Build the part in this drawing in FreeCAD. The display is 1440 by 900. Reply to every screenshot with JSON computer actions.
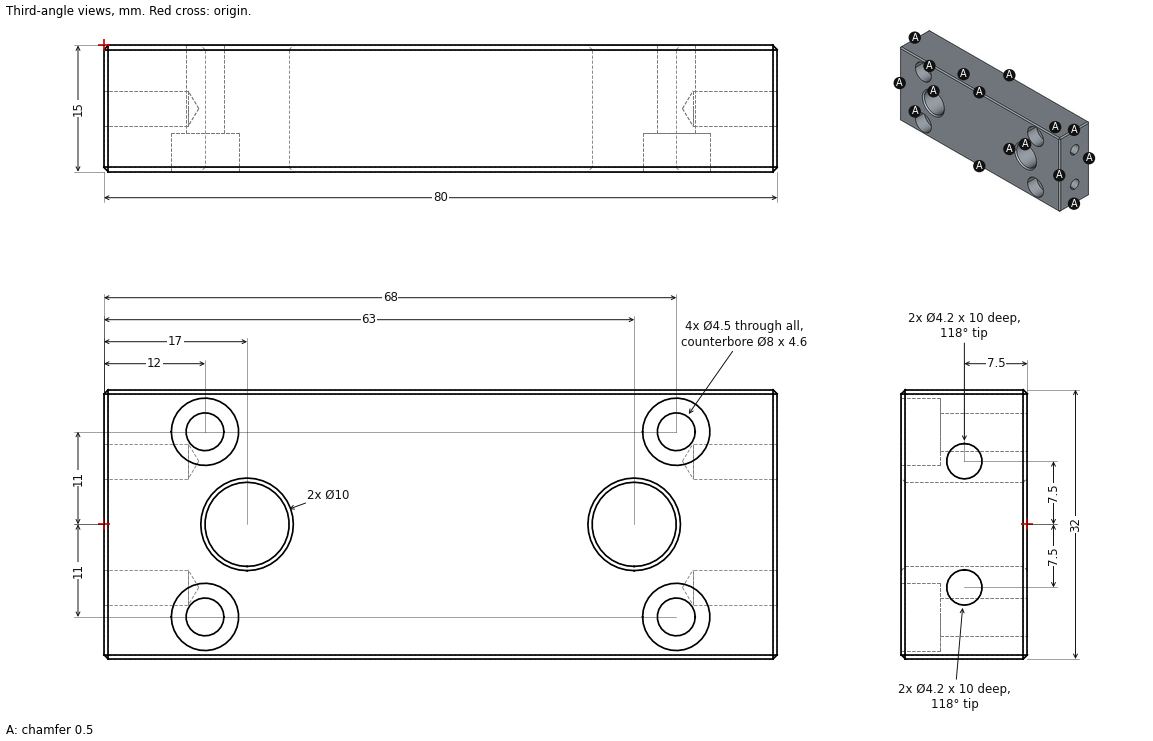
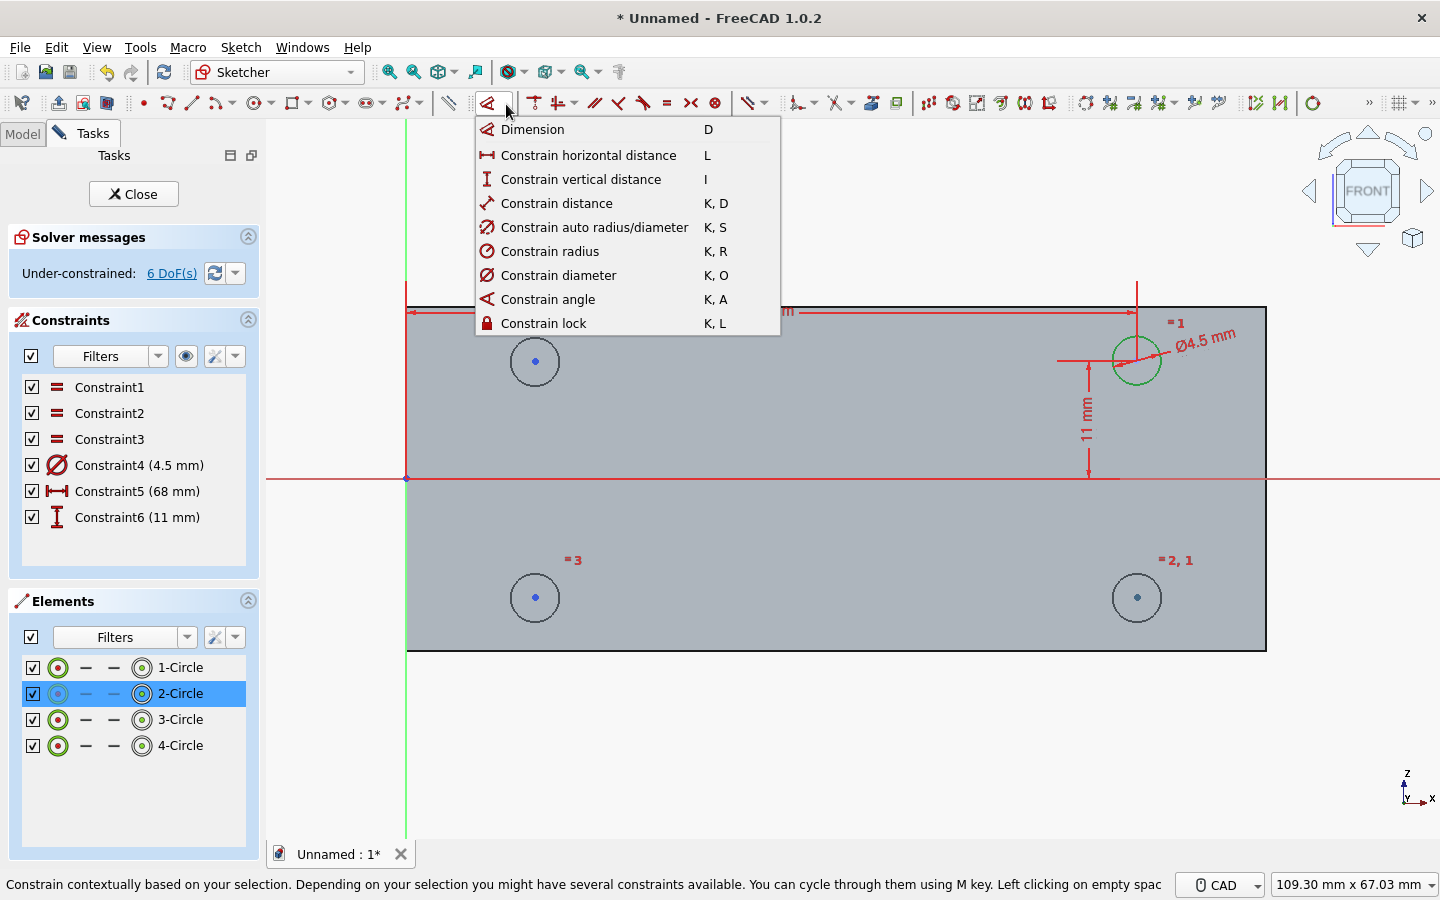
{"action": "left_click", "coordinate": [628, 155]}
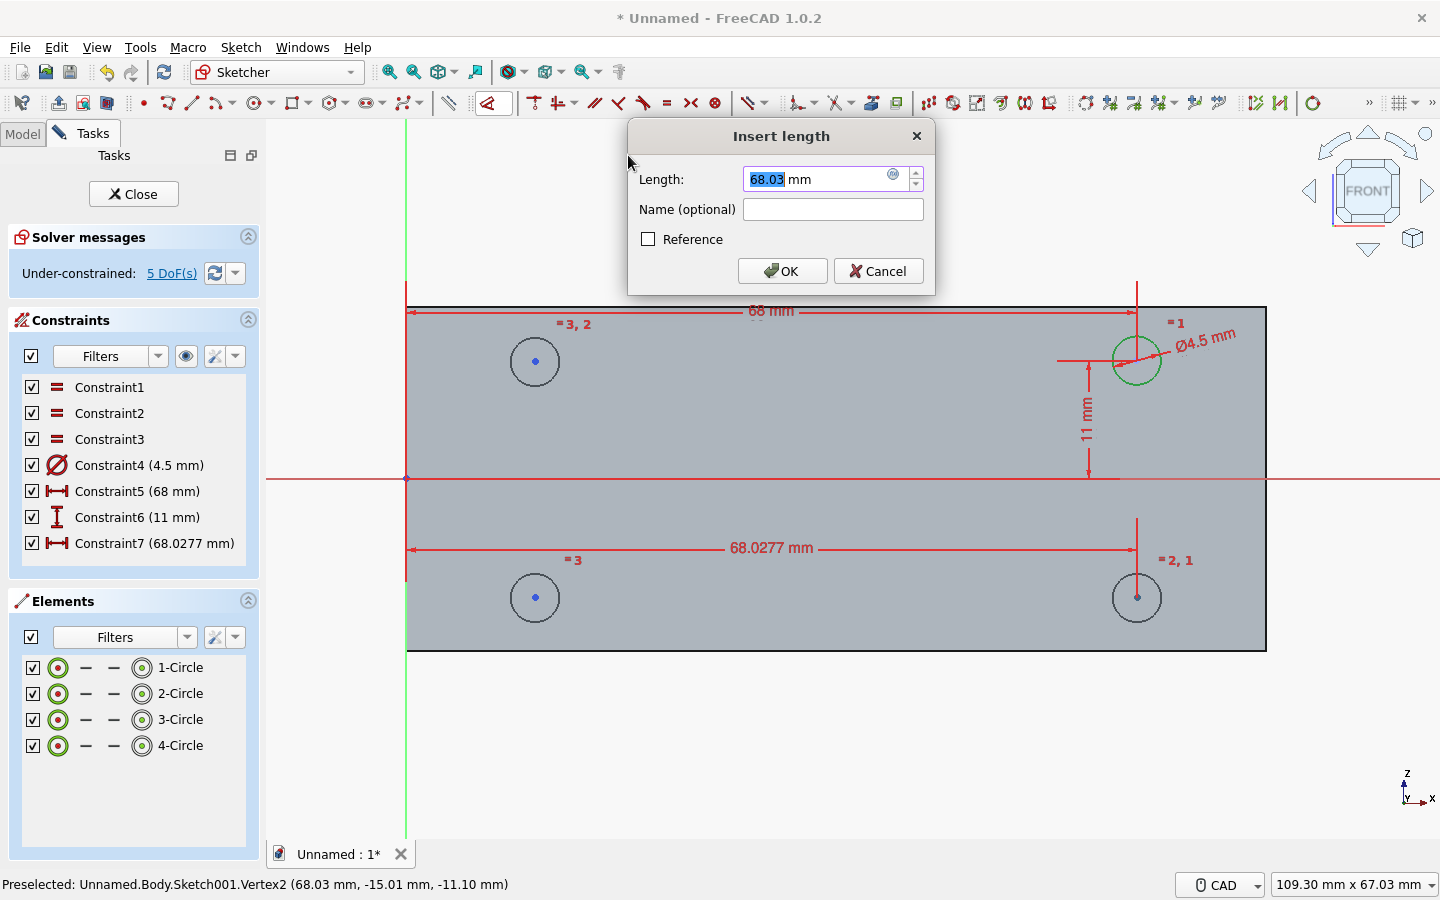
{"action": "type", "text": "68"}
{"action": "key", "text": "Return"}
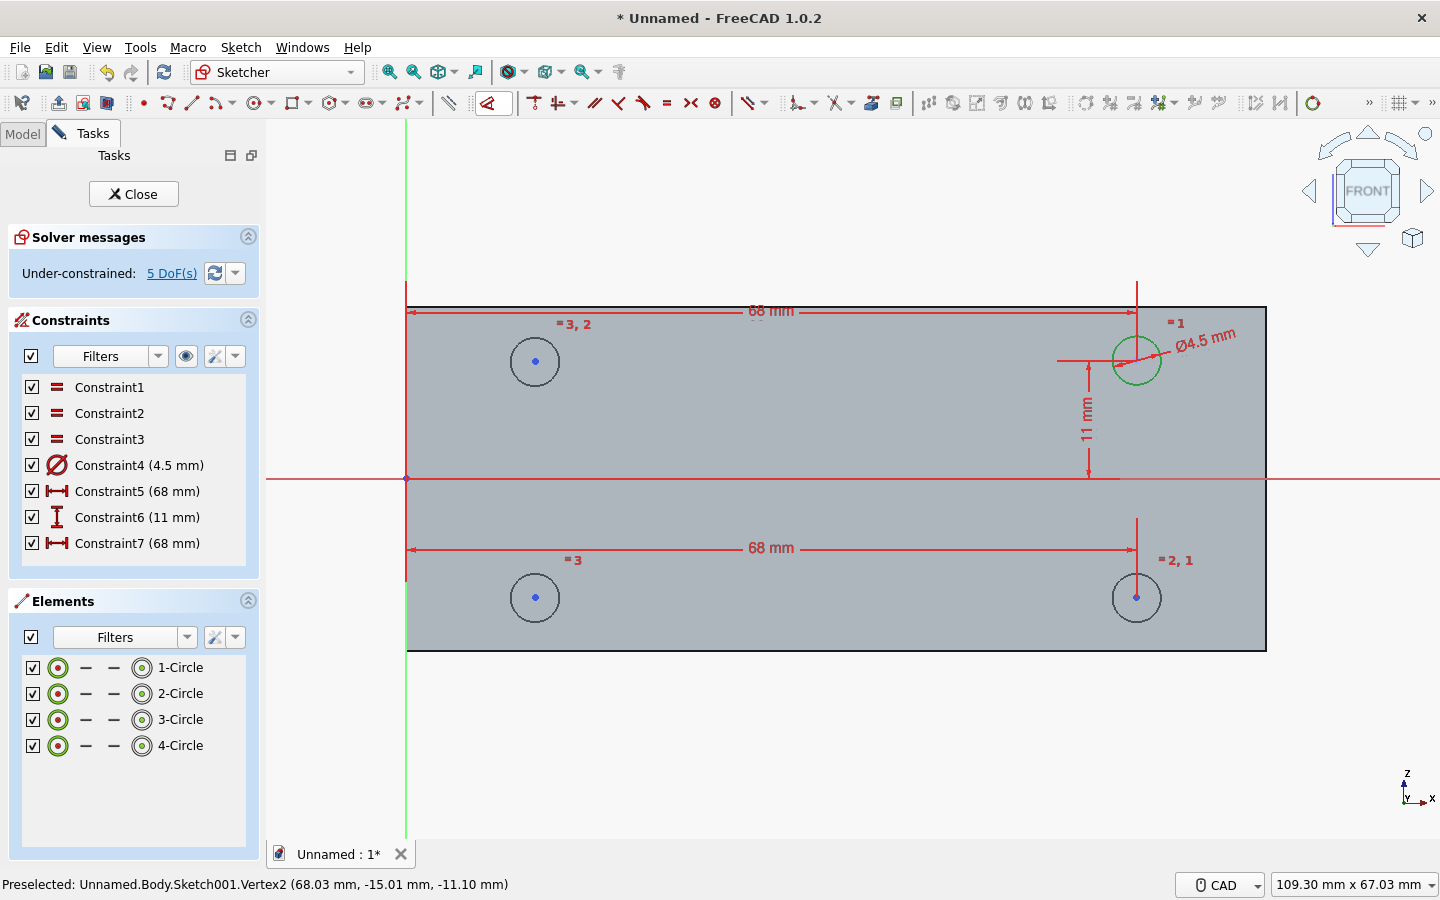
{"action": "left_click", "coordinate": [1137, 598]}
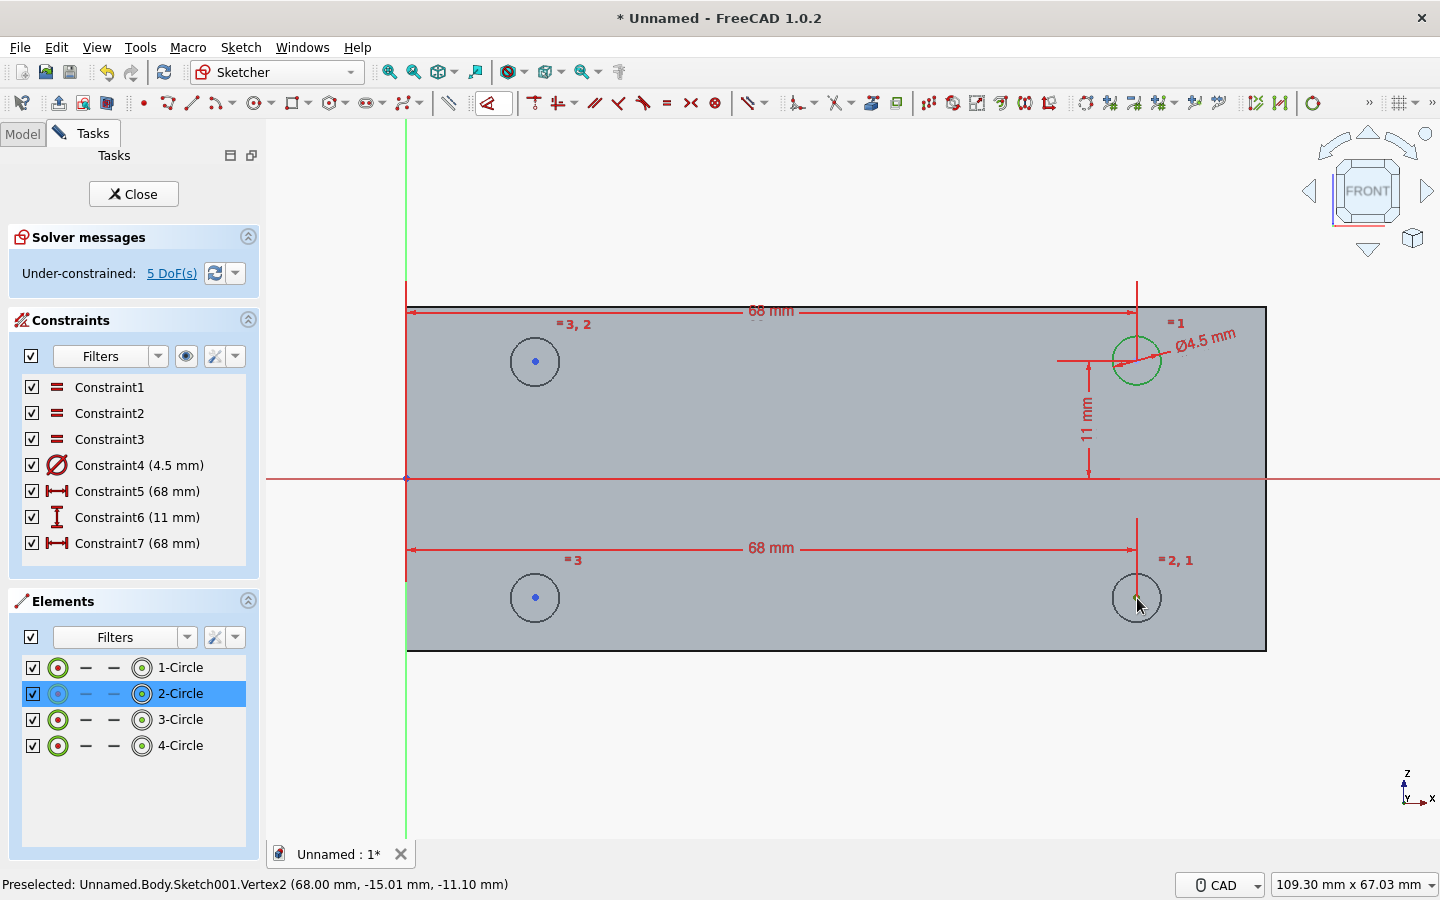
{"action": "left_click", "coordinate": [506, 104]}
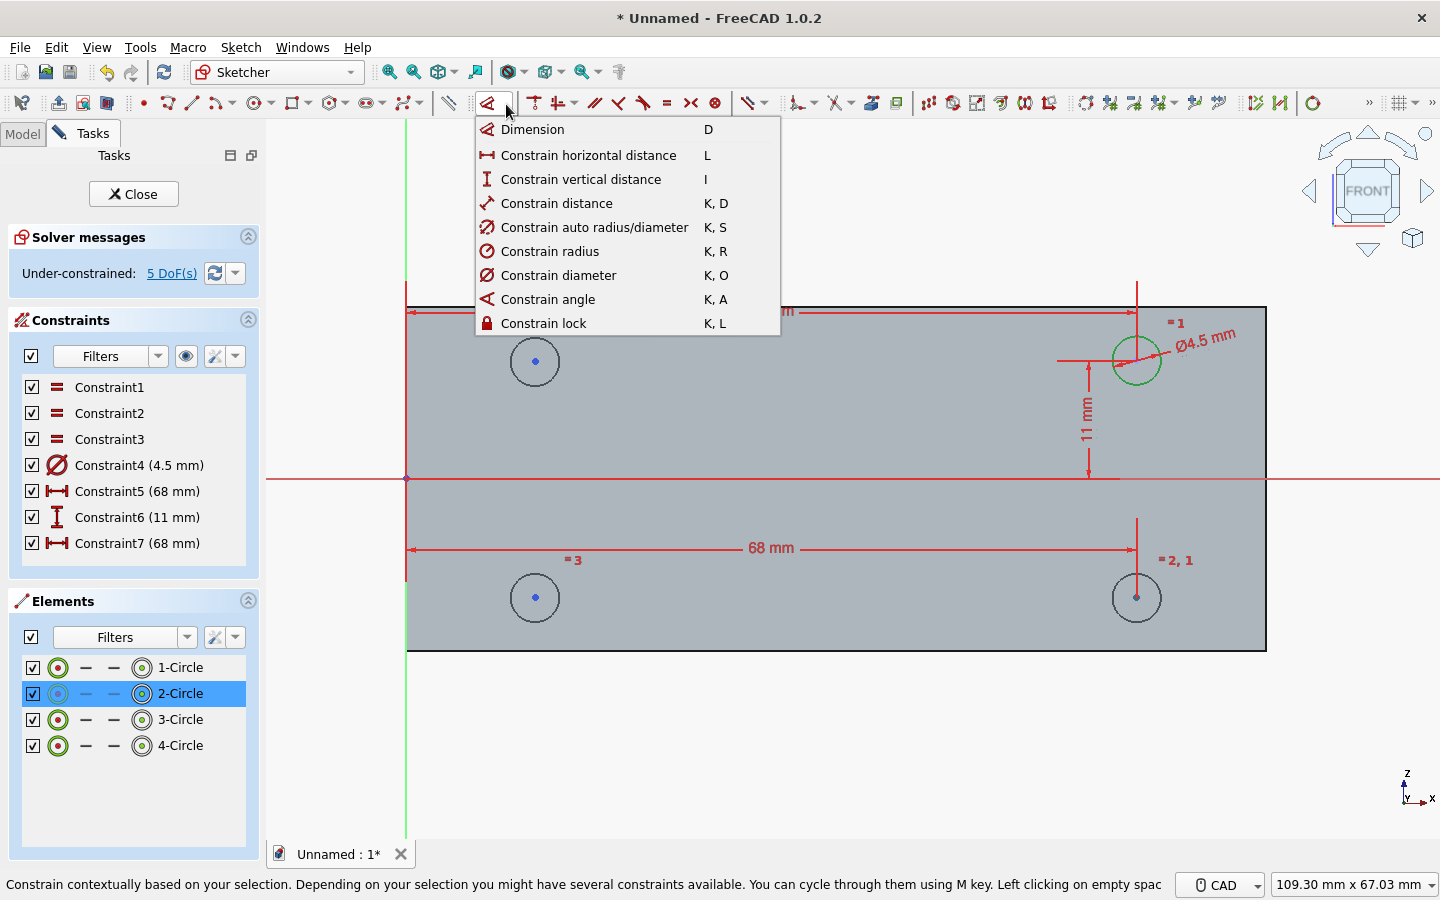
{"action": "left_click", "coordinate": [628, 179]}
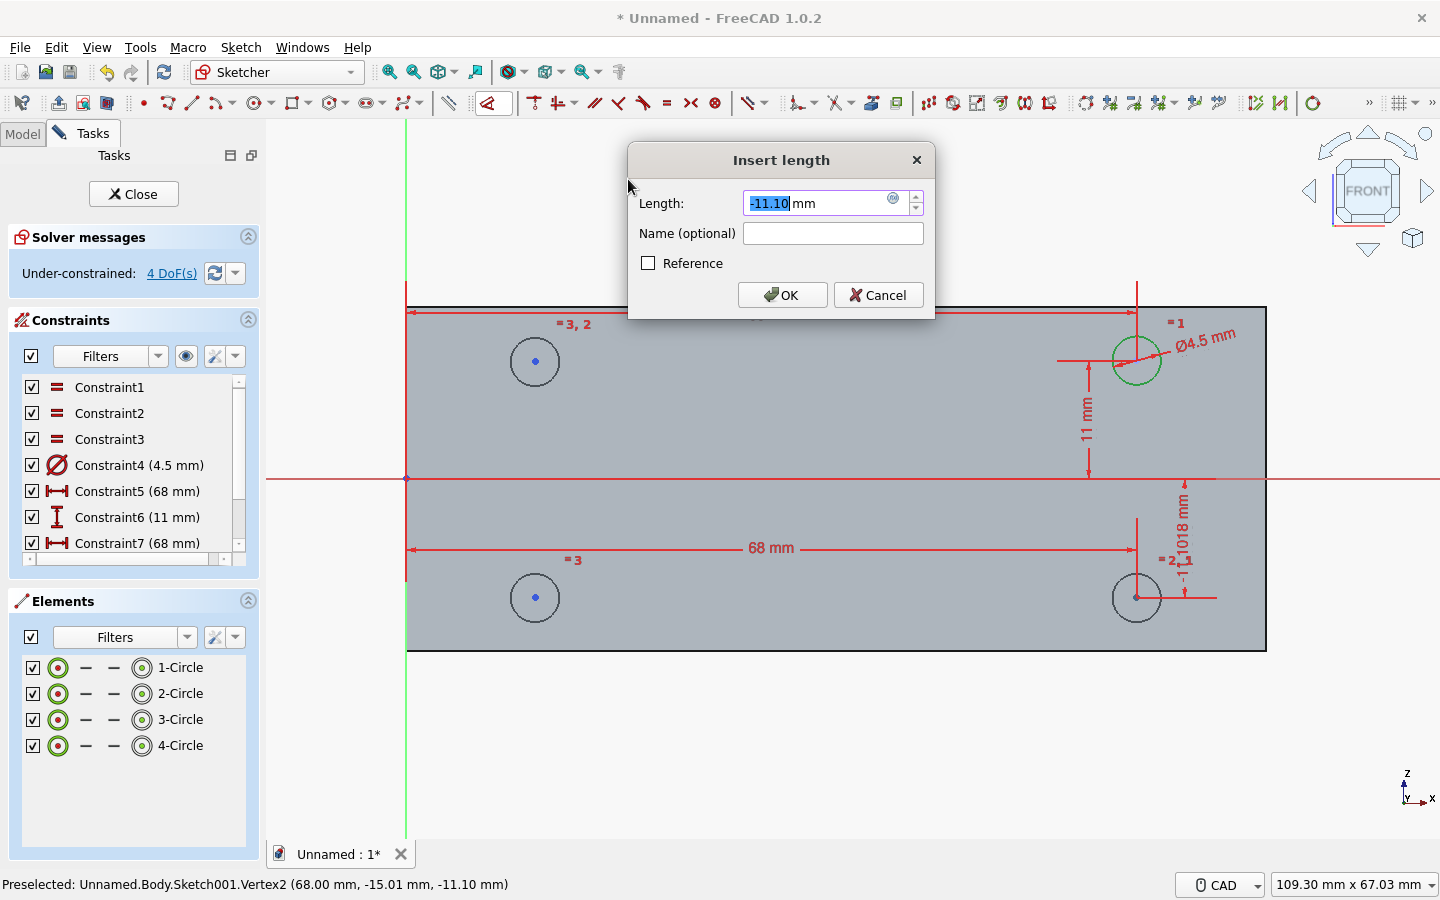
{"action": "type", "text": "-11"}
{"action": "key", "text": "Return"}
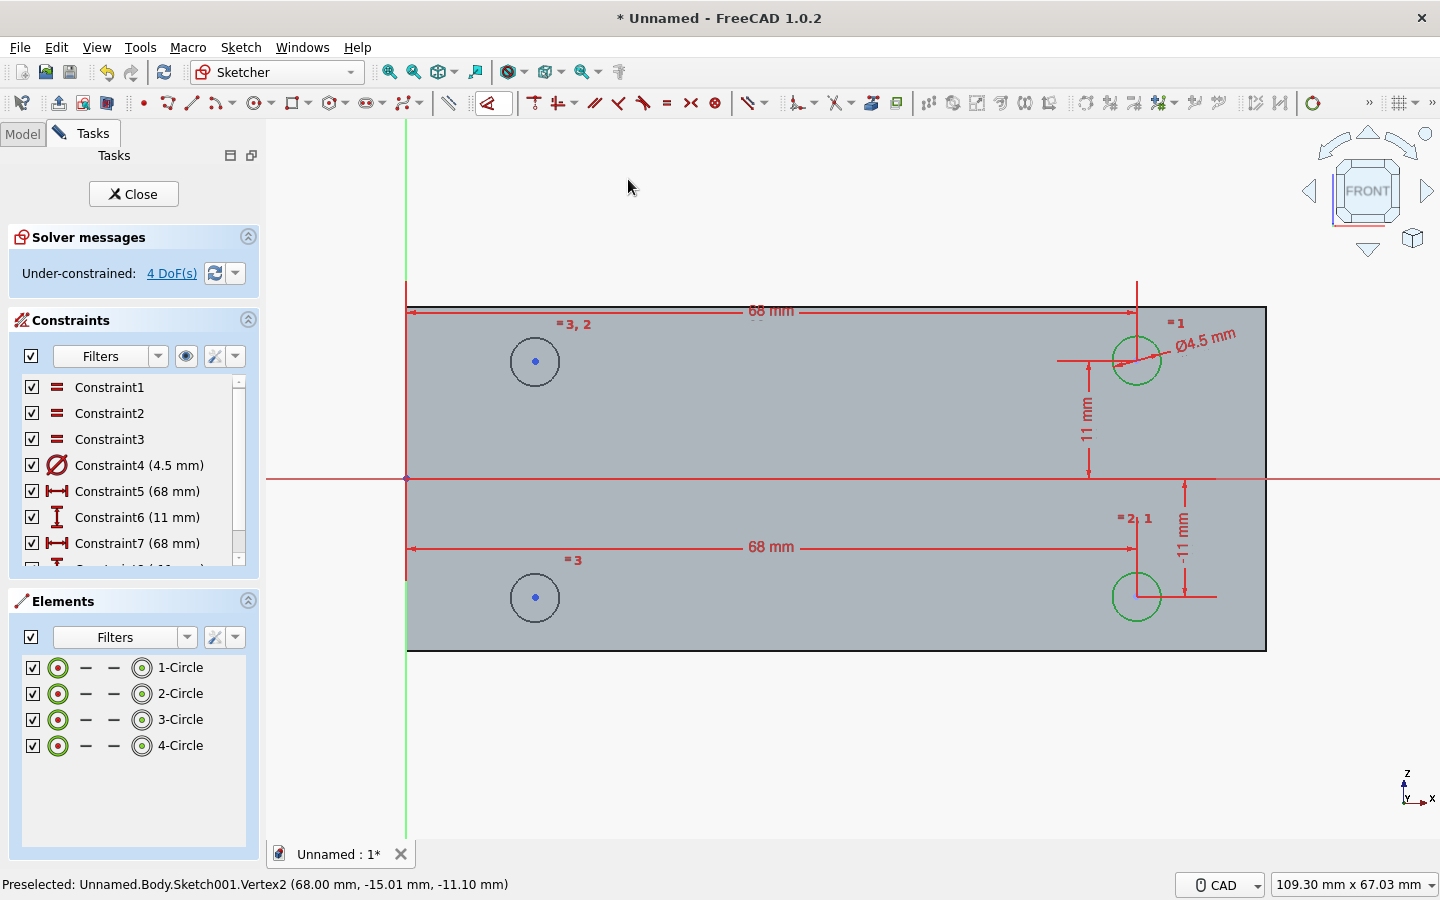
{"action": "left_click", "coordinate": [535, 362]}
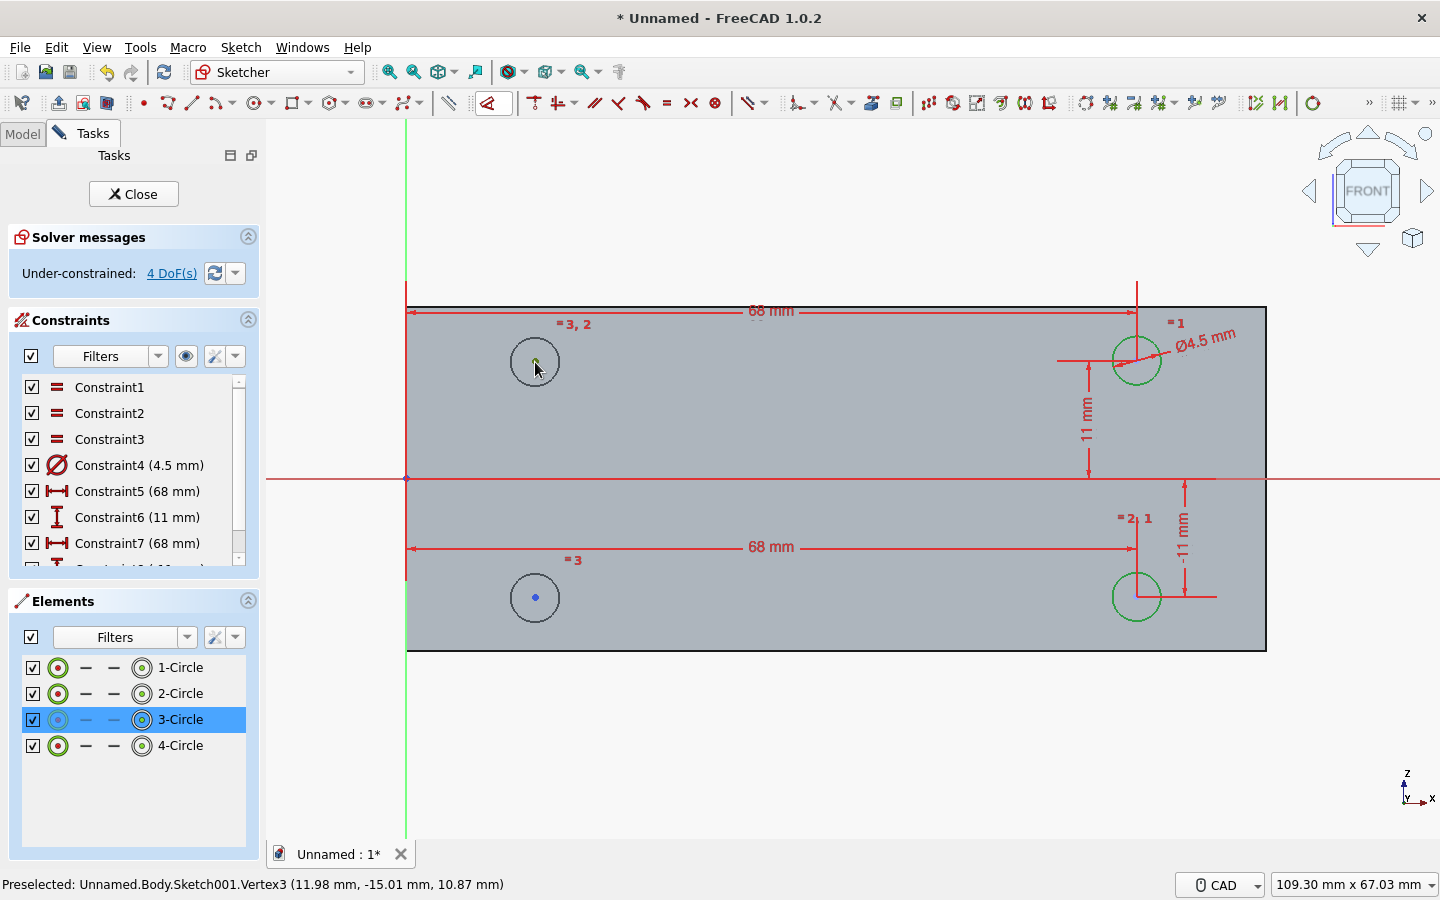
{"action": "key", "text": "l"}